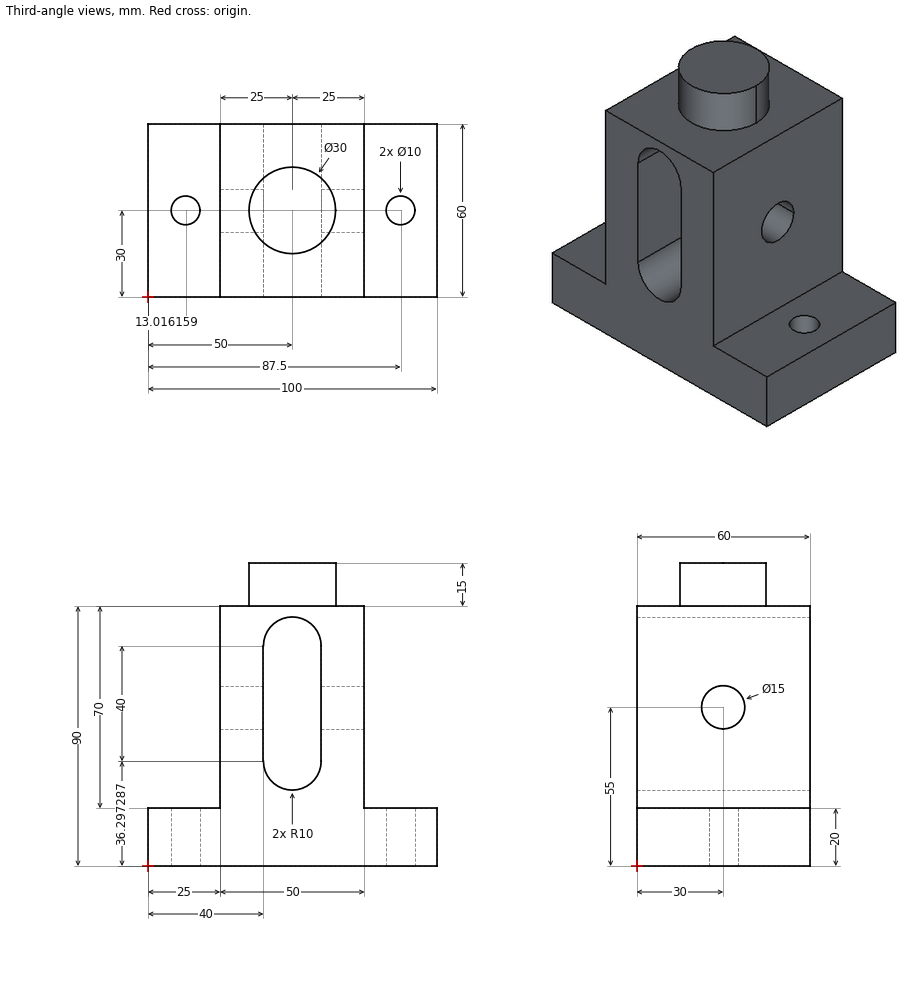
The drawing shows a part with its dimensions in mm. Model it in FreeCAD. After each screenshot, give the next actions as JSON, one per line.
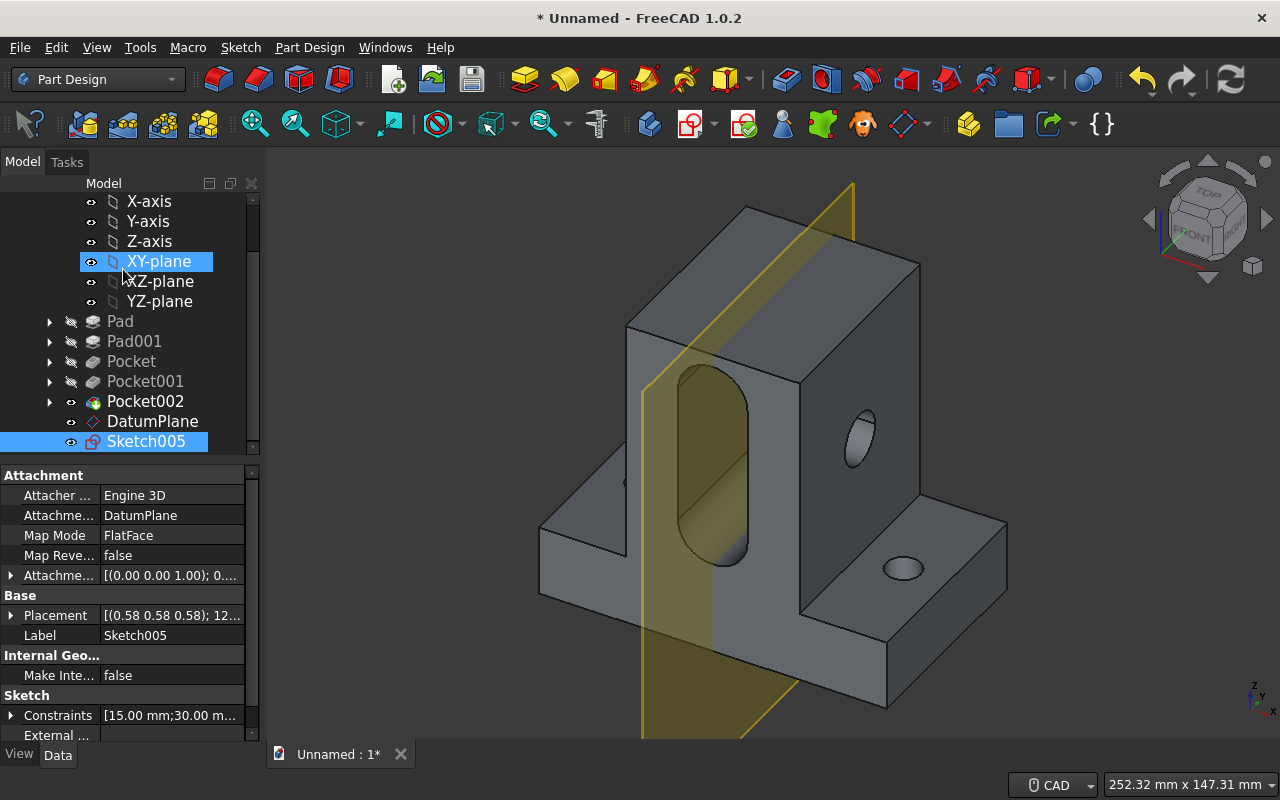
{"action": "left_click", "coordinate": [788, 80]}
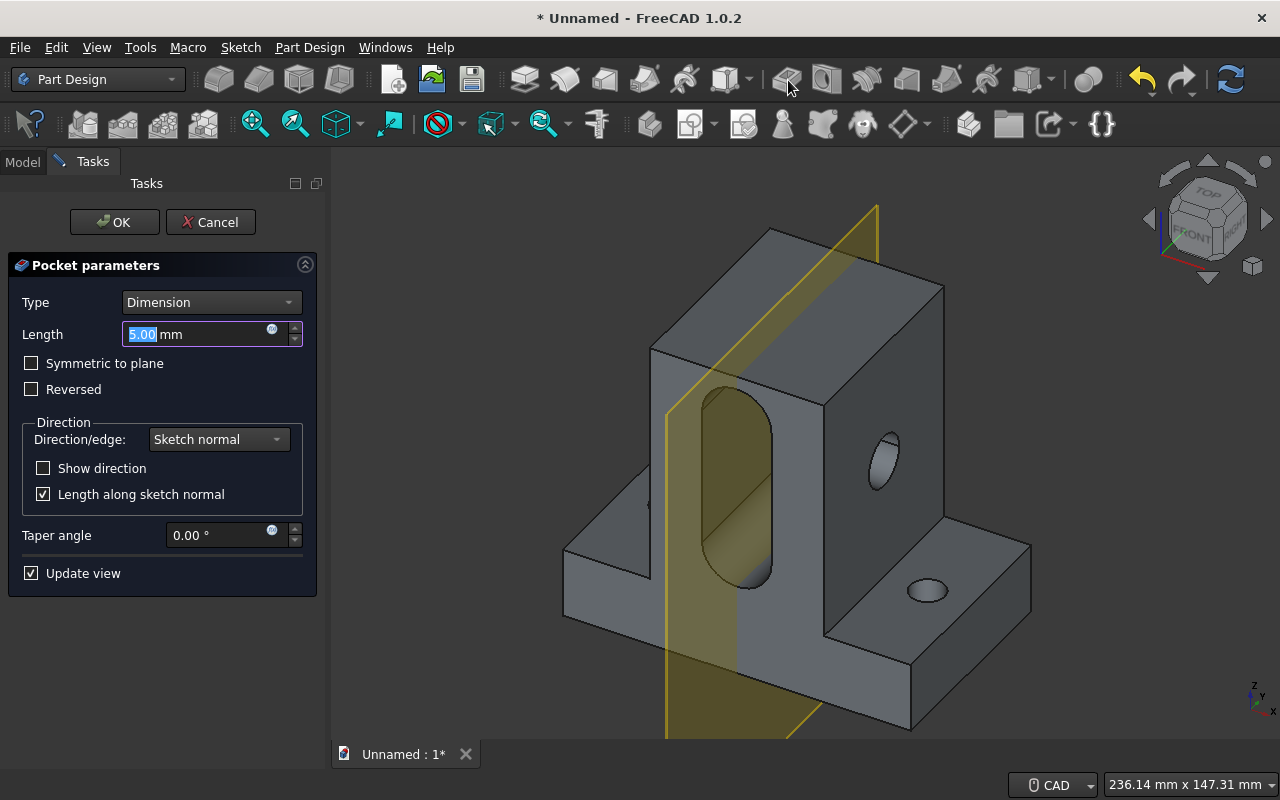
{"action": "type", "text": "25"}
{"action": "key", "text": "Tab"}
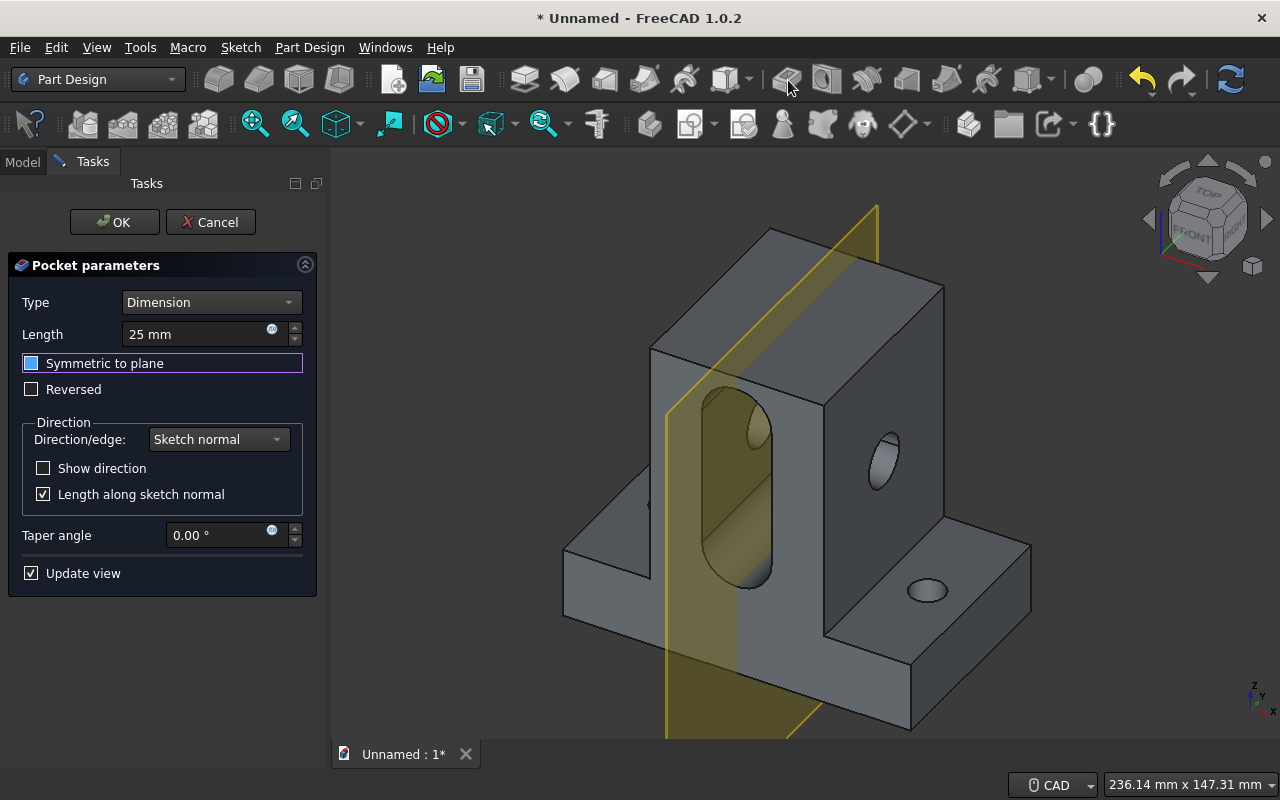
{"action": "left_click", "coordinate": [115, 222]}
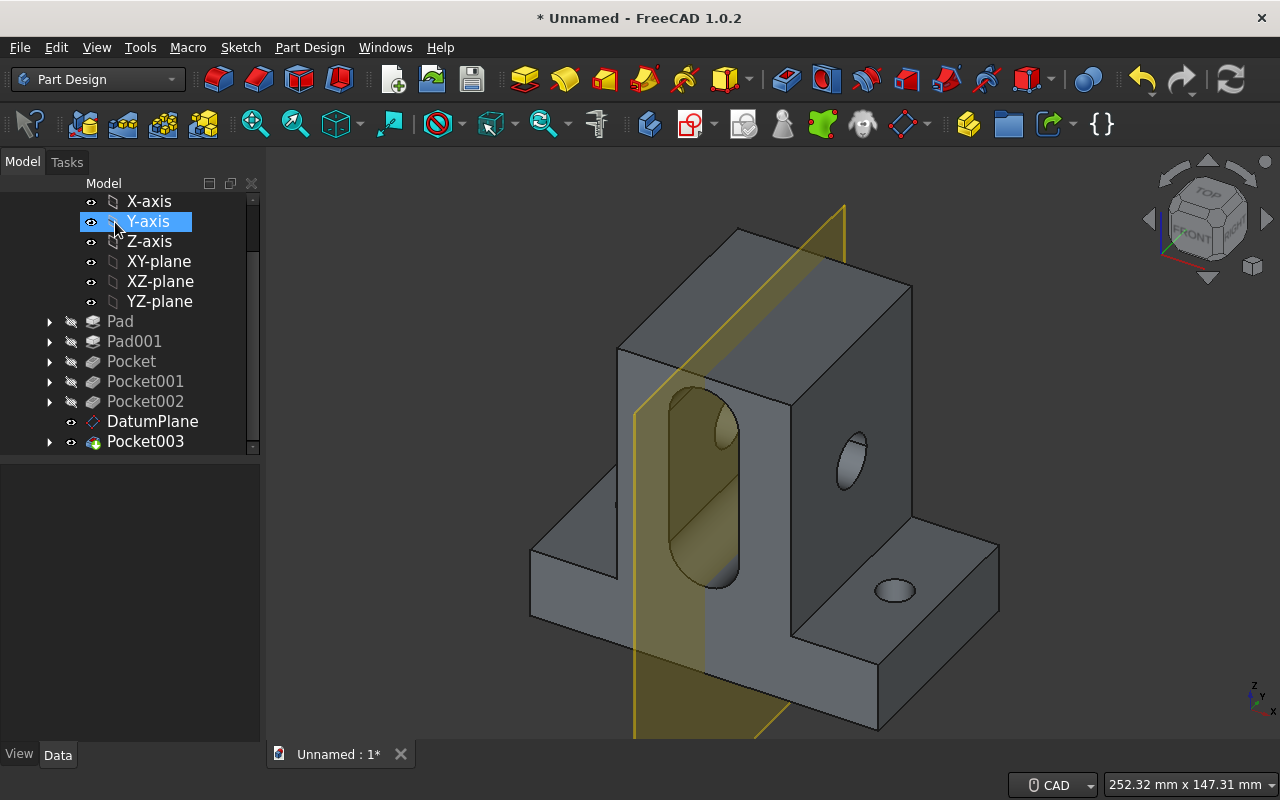
{"action": "left_click", "coordinate": [116, 422]}
{"action": "key", "text": "space"}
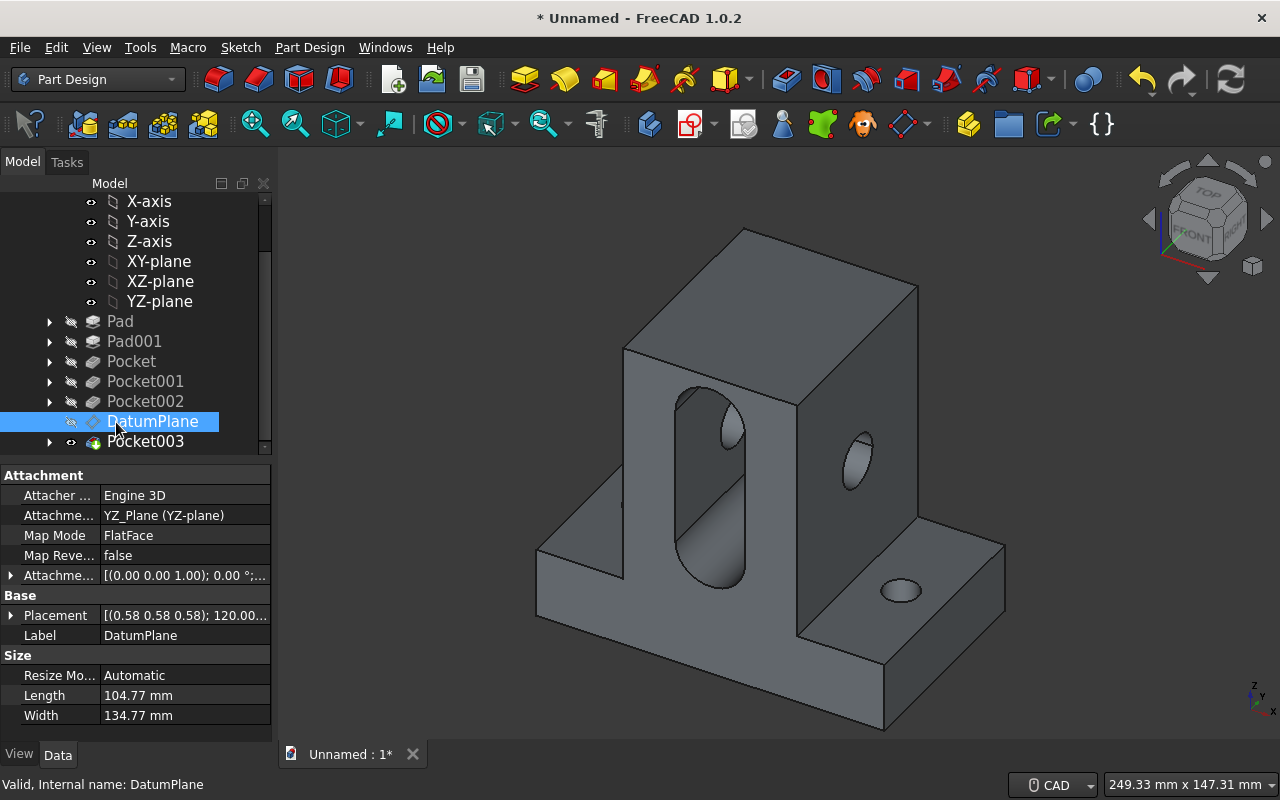
{"action": "left_click", "coordinate": [771, 316]}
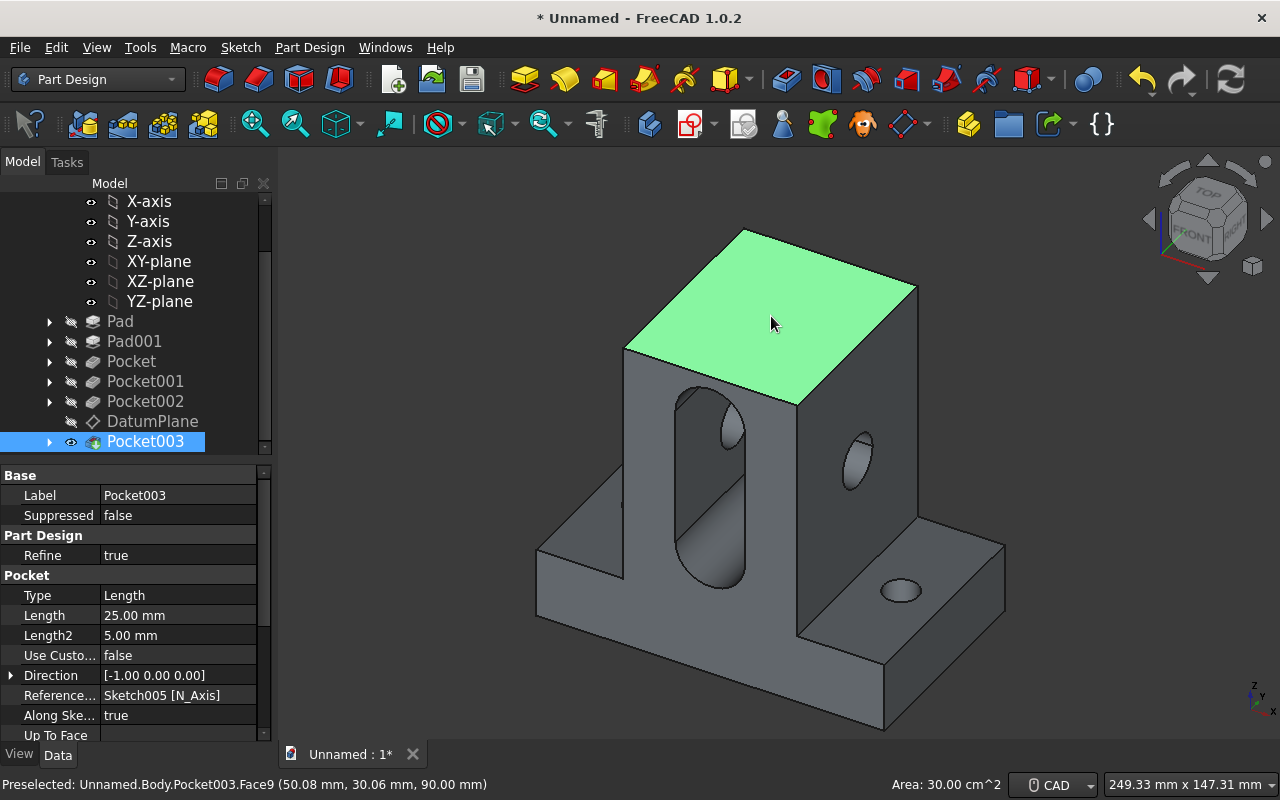
{"action": "left_click", "coordinate": [690, 124]}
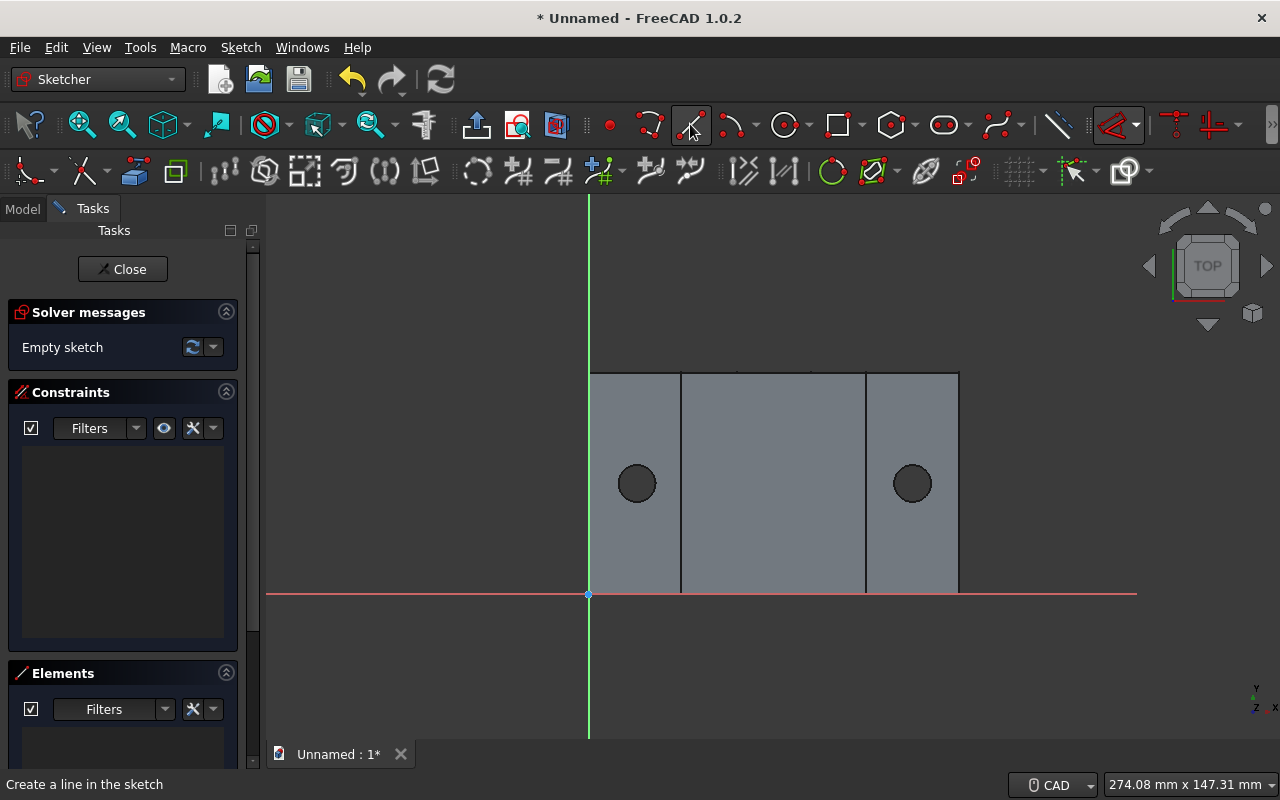
{"action": "scroll", "coordinate": [713, 548], "scroll_direction": "up", "scroll_amount": 4}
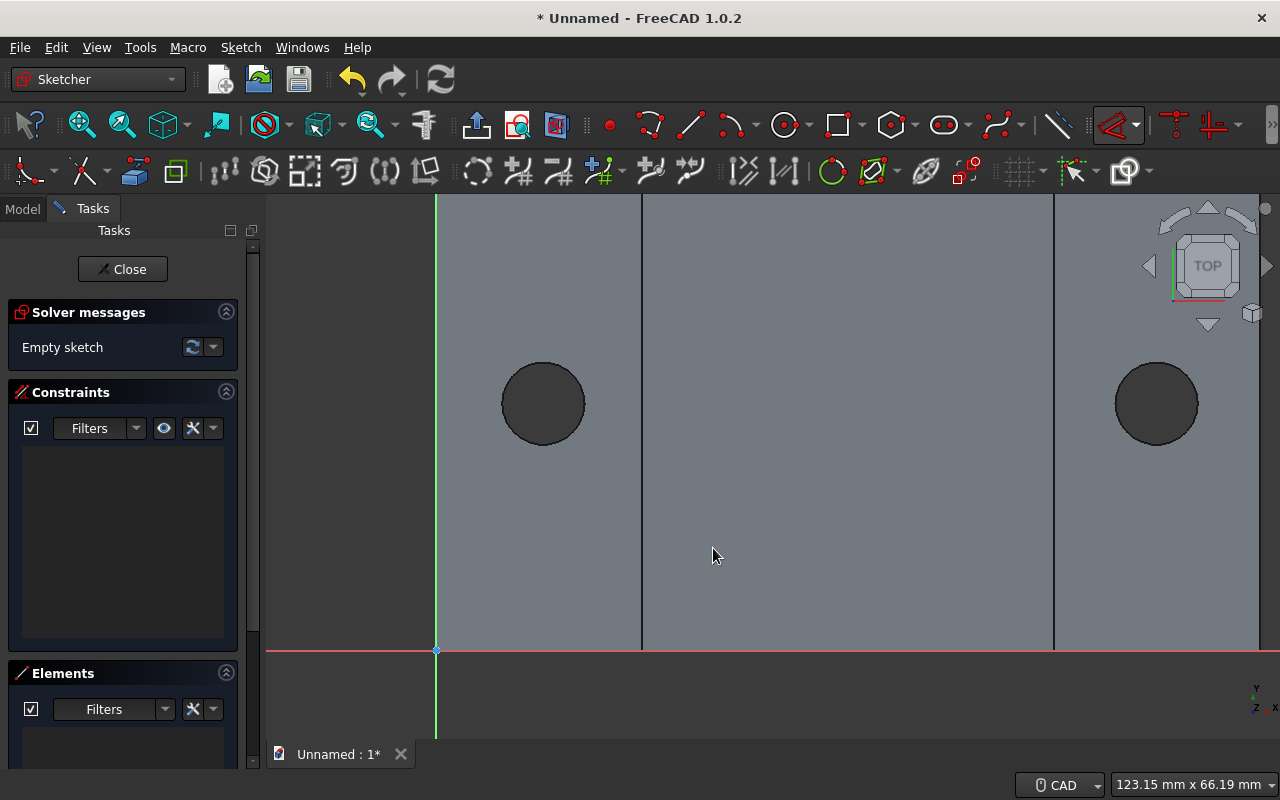
{"action": "key", "text": "g c"}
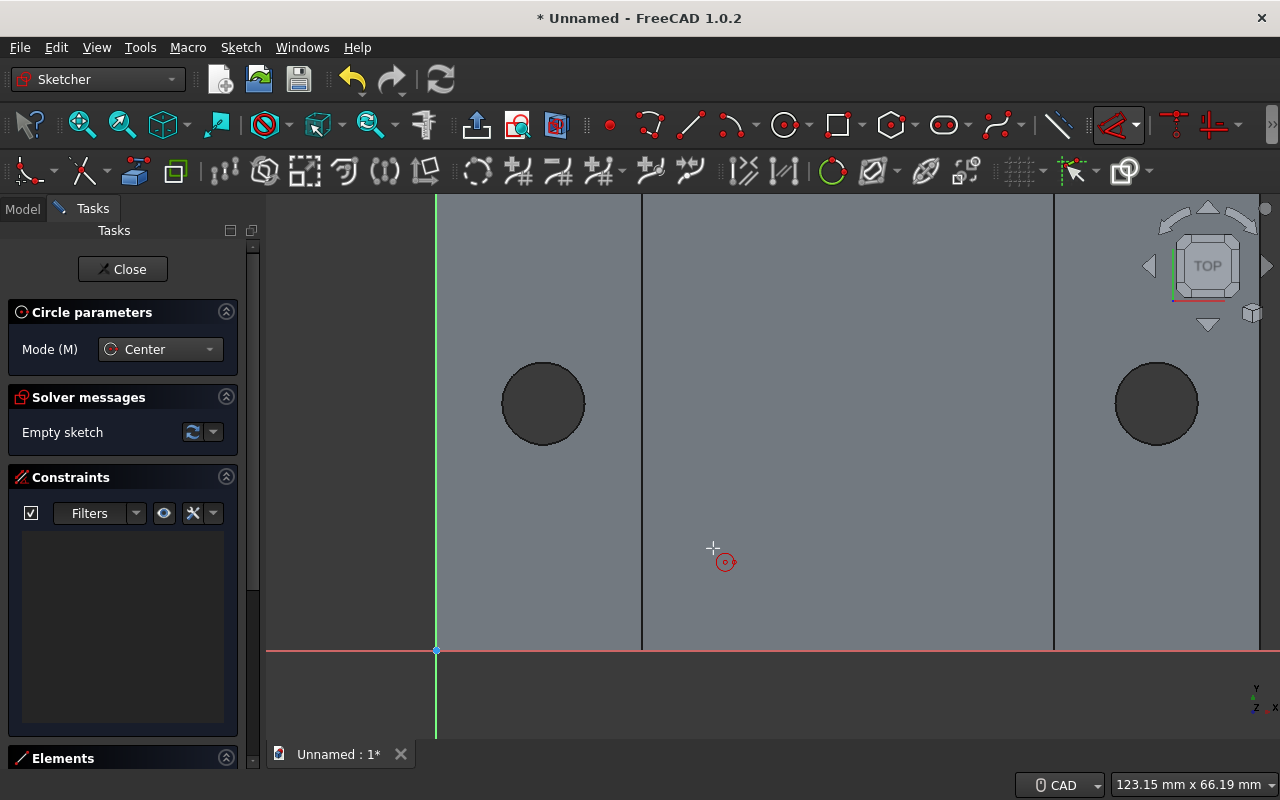
{"action": "left_click", "coordinate": [848, 404]}
{"action": "left_click", "coordinate": [935, 316]}
{"action": "key", "text": "Escape"}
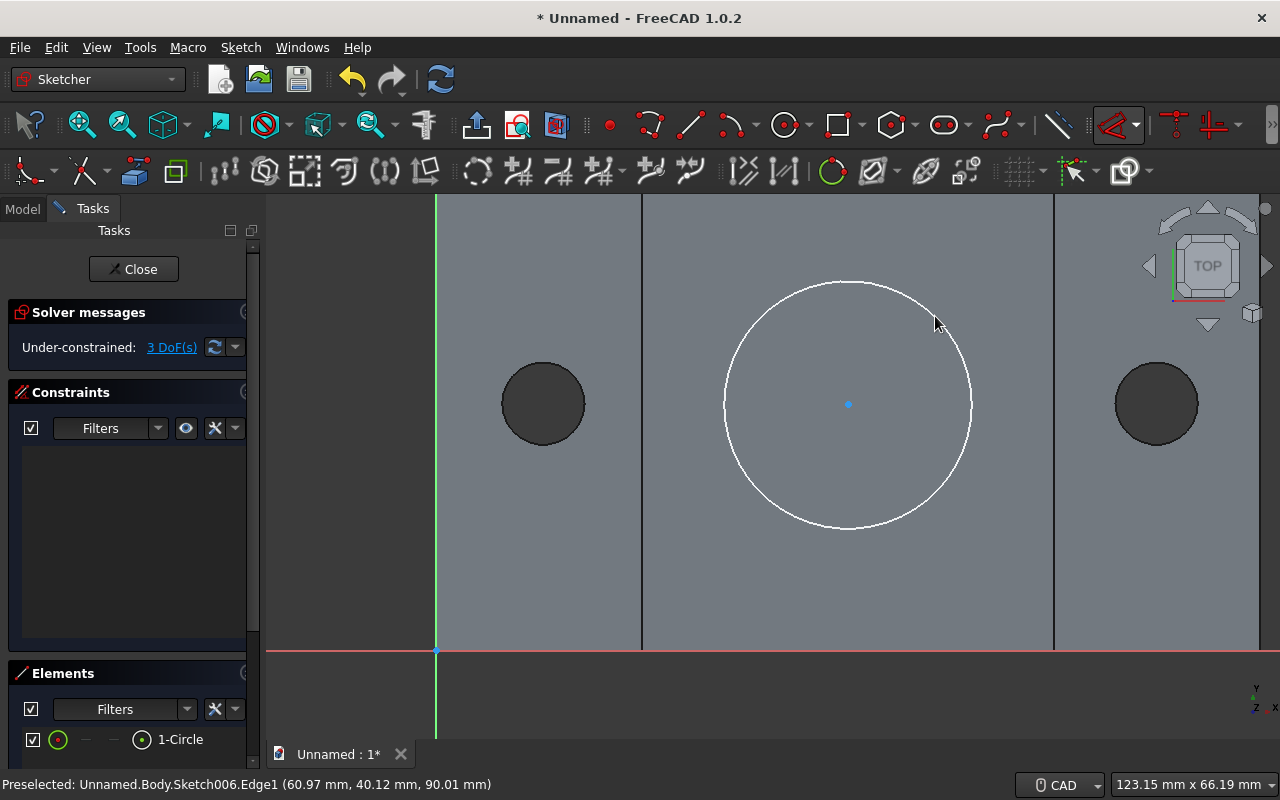
{"action": "left_click", "coordinate": [935, 317]}